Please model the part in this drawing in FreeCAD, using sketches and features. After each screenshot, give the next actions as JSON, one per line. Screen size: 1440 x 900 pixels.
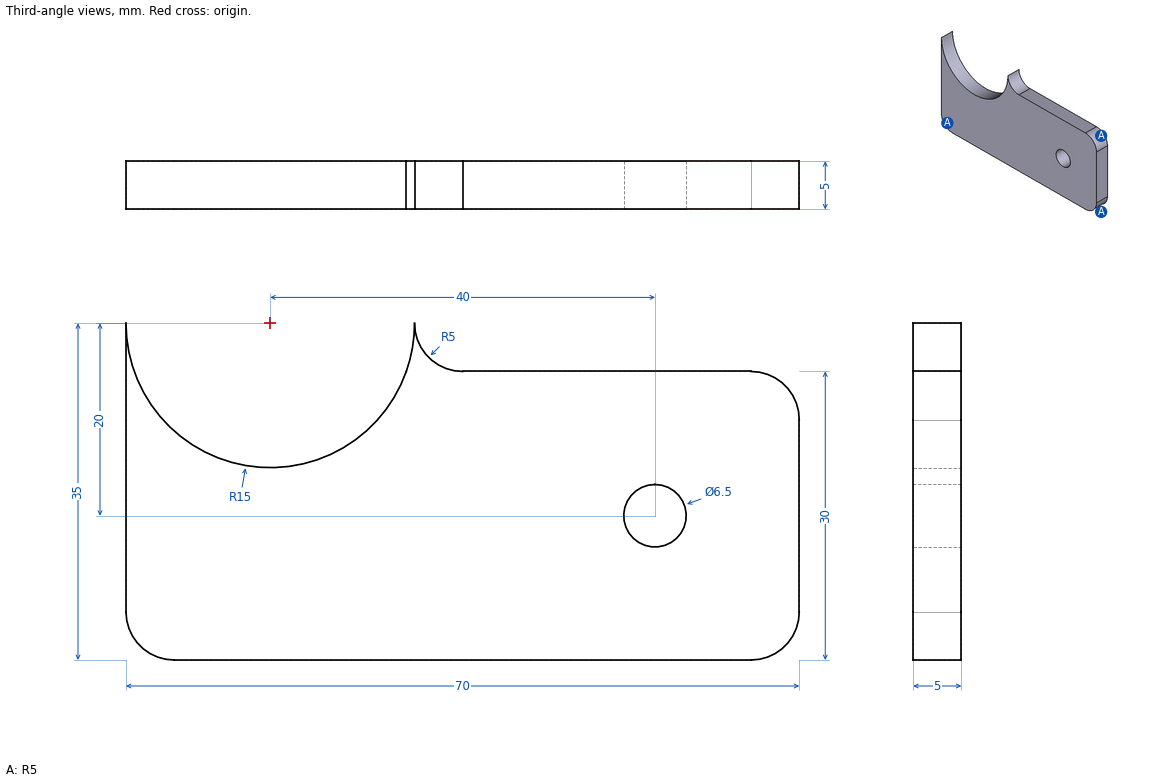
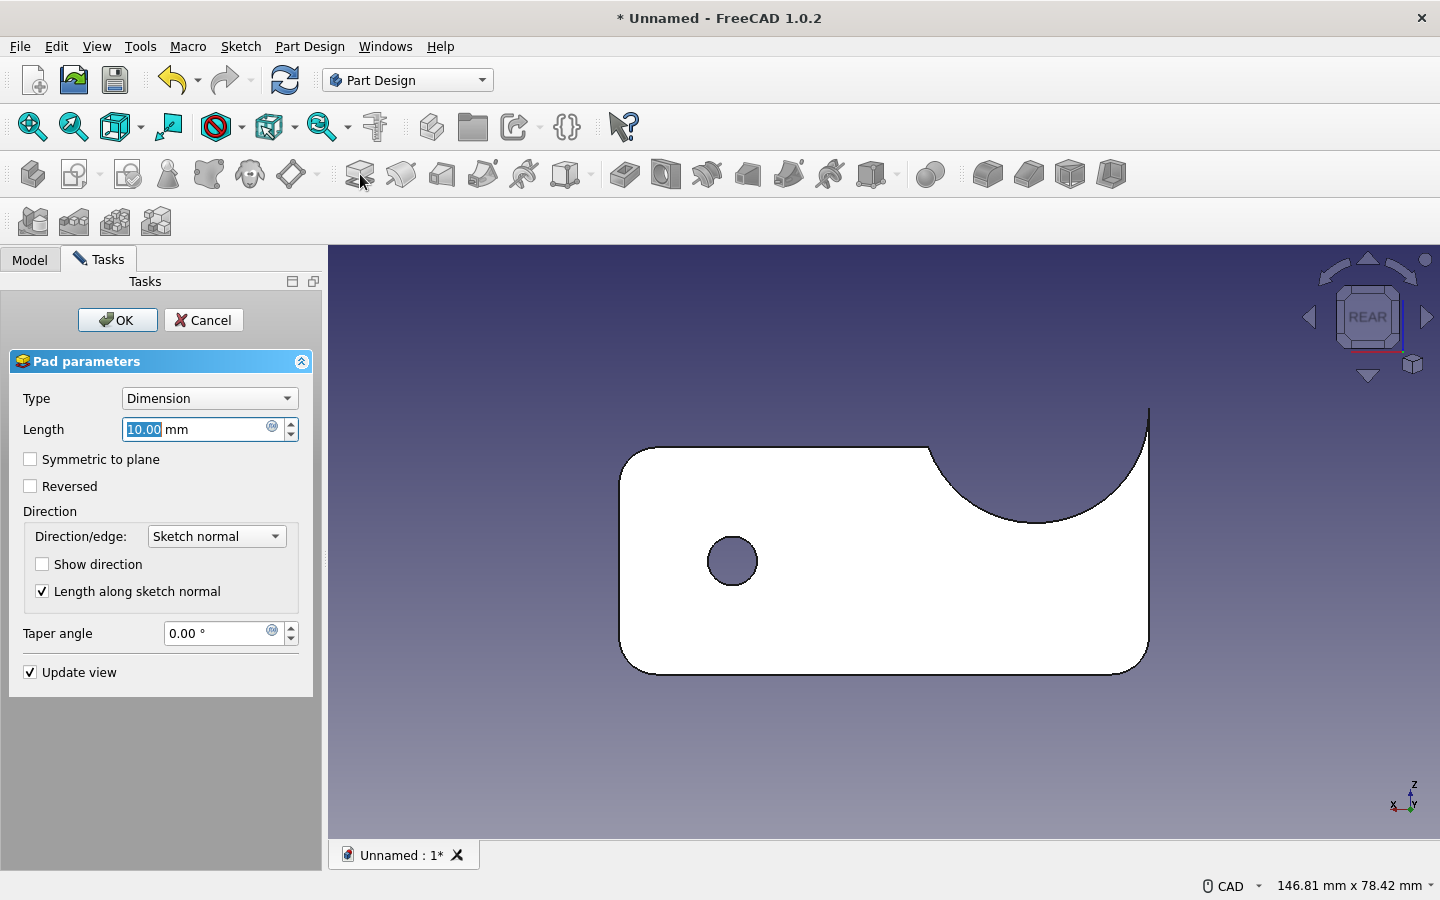
{"action": "type", "text": "5"}
{"action": "key", "text": "Tab"}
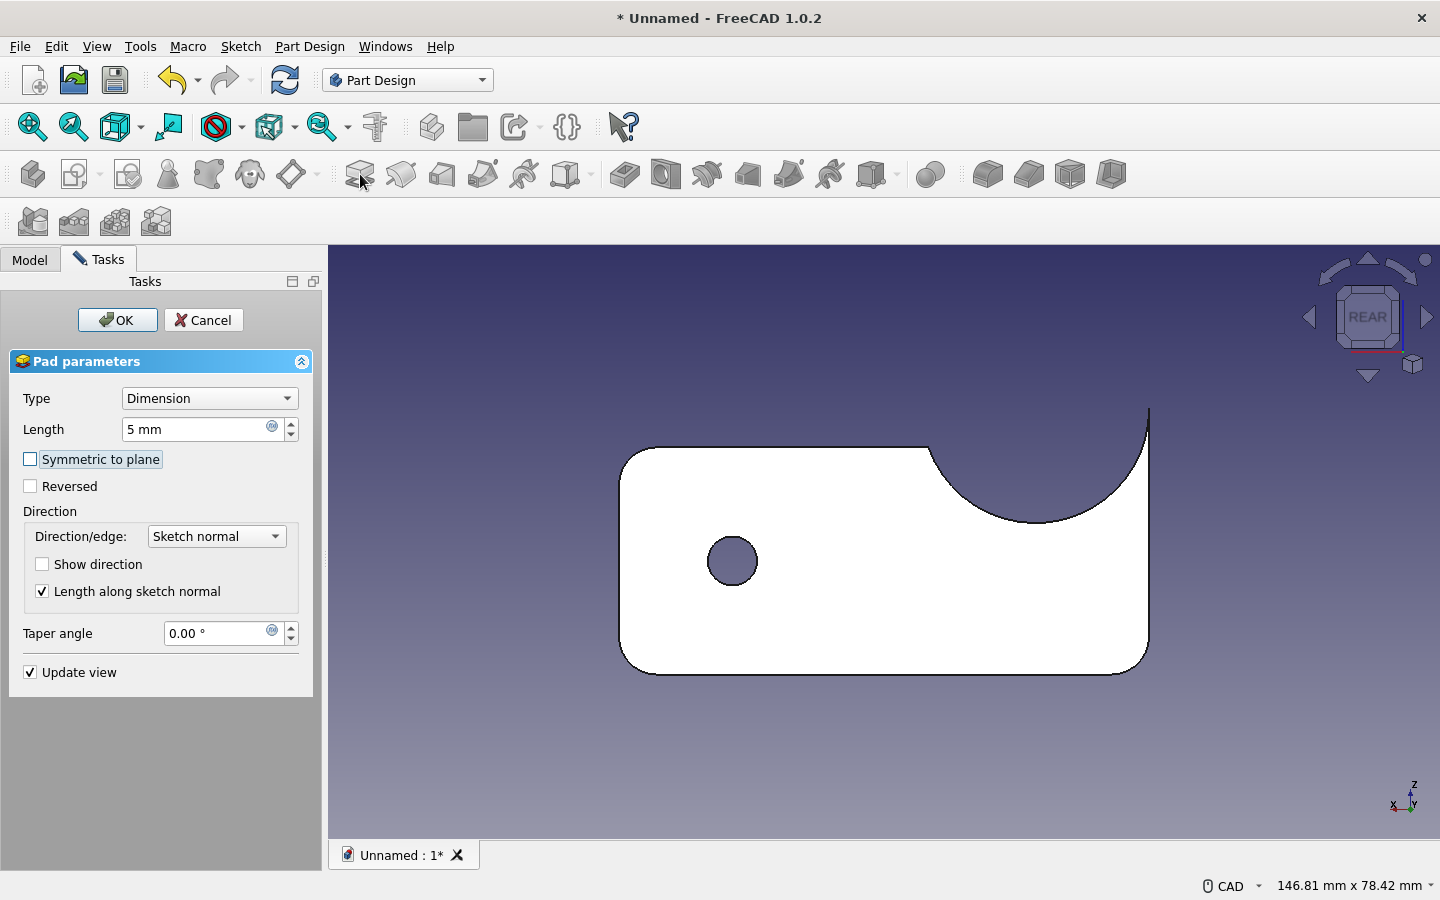
{"action": "left_click", "coordinate": [31, 486]}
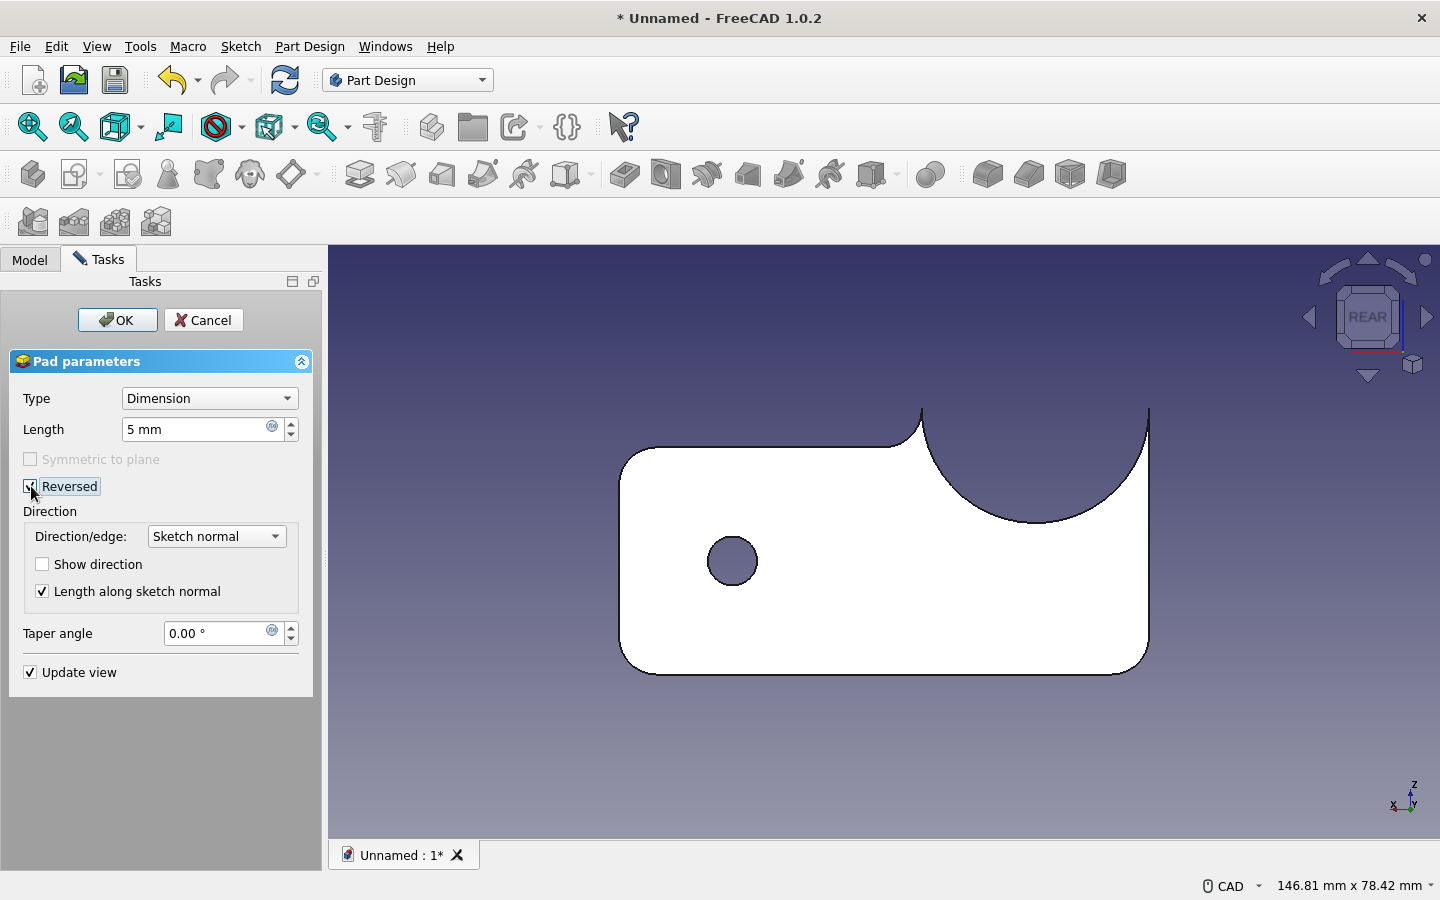
{"action": "left_click", "coordinate": [118, 320]}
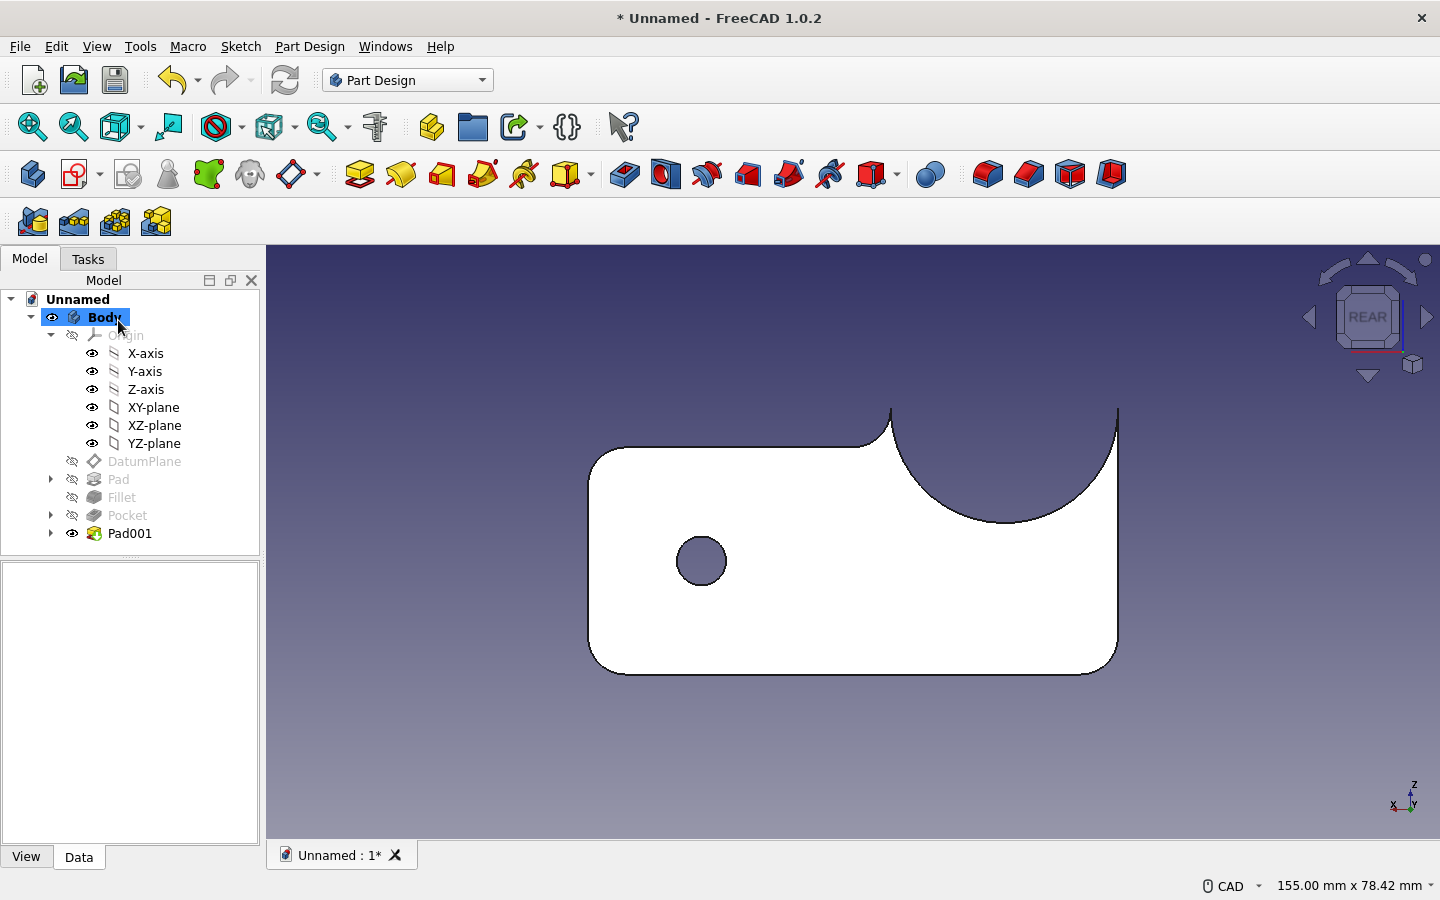
{"action": "key", "text": "0"}